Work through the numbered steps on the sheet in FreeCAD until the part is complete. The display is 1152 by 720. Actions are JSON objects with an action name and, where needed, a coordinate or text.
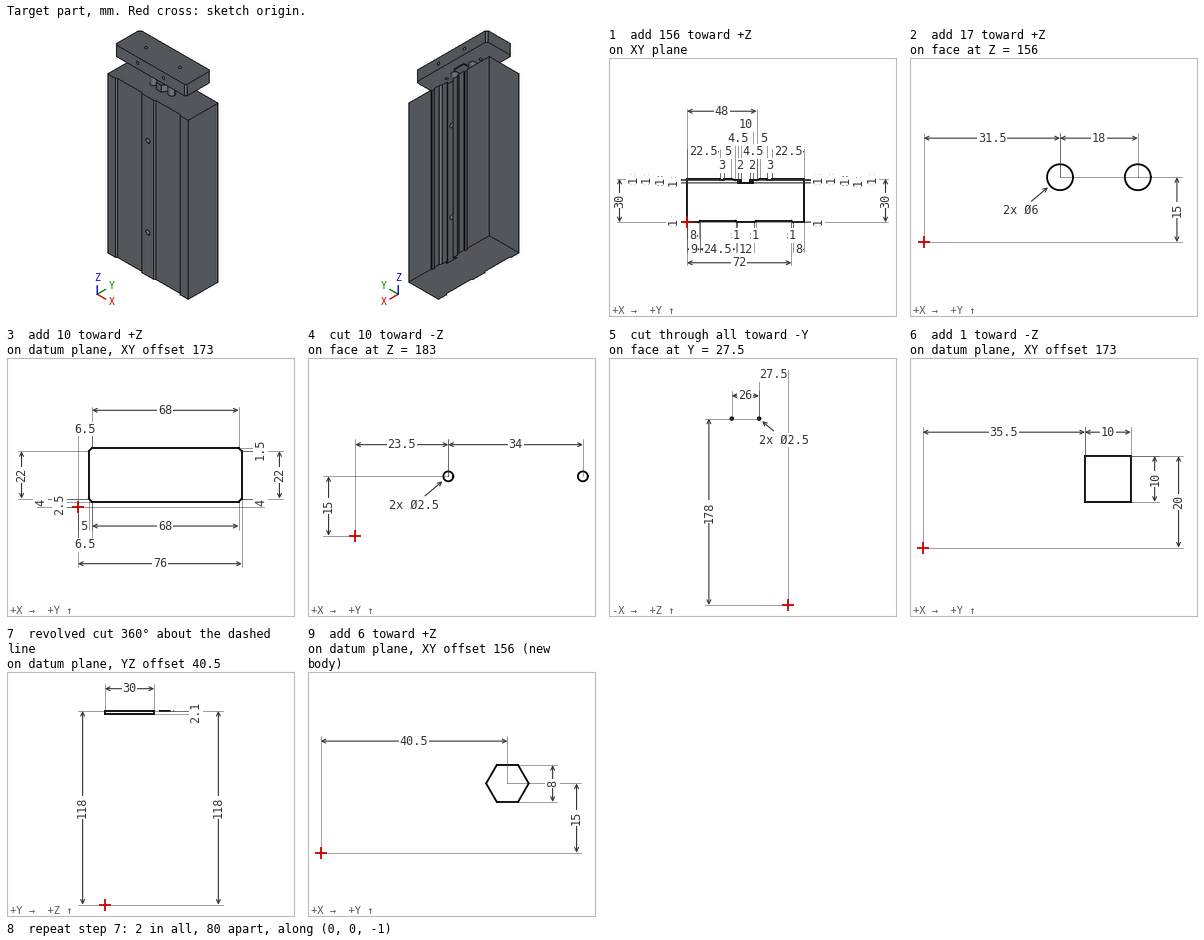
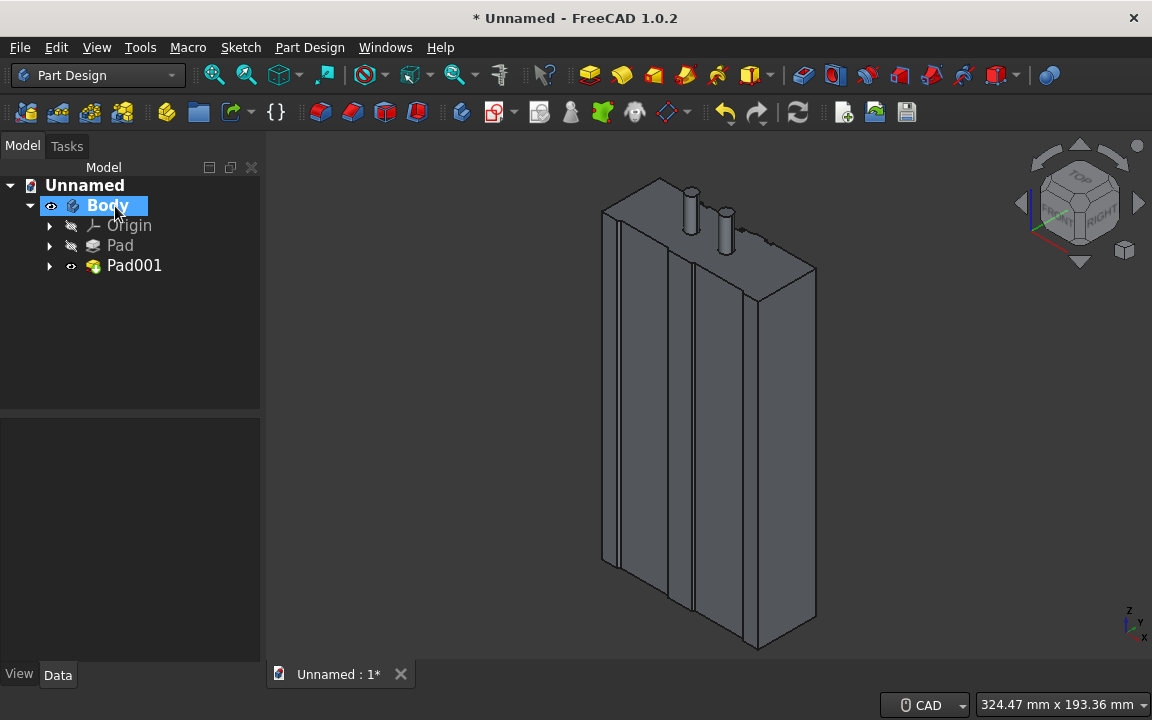
{"action": "key", "text": "2"}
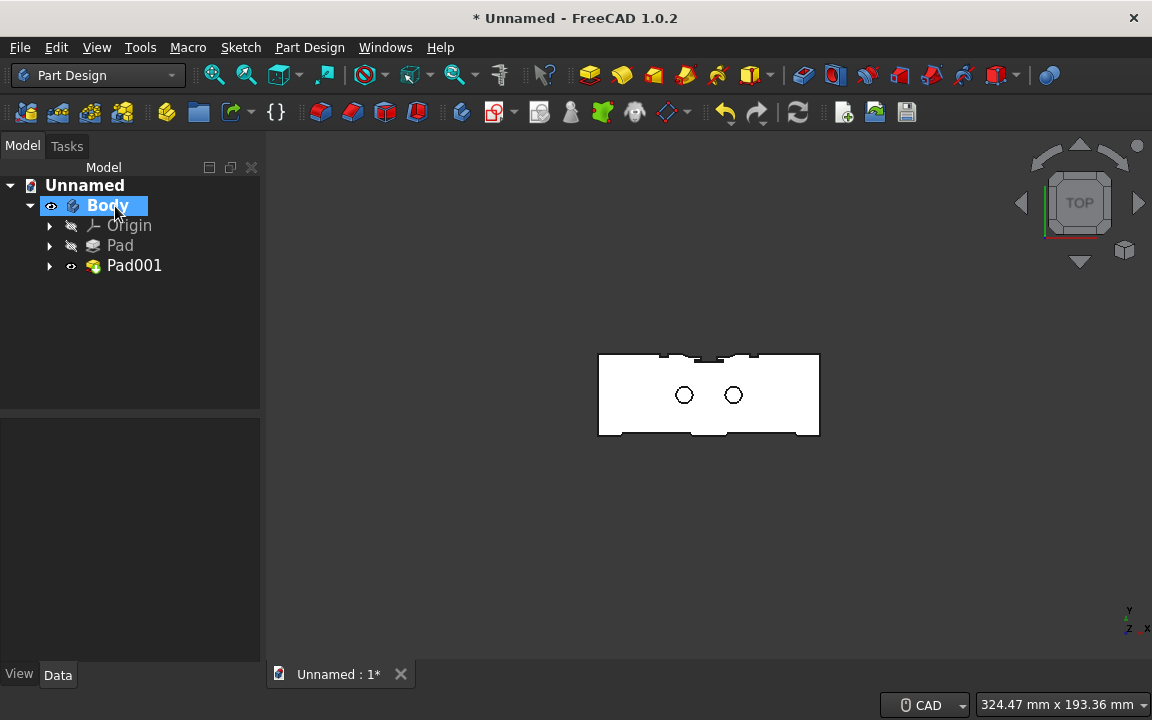
{"action": "key", "text": "v f"}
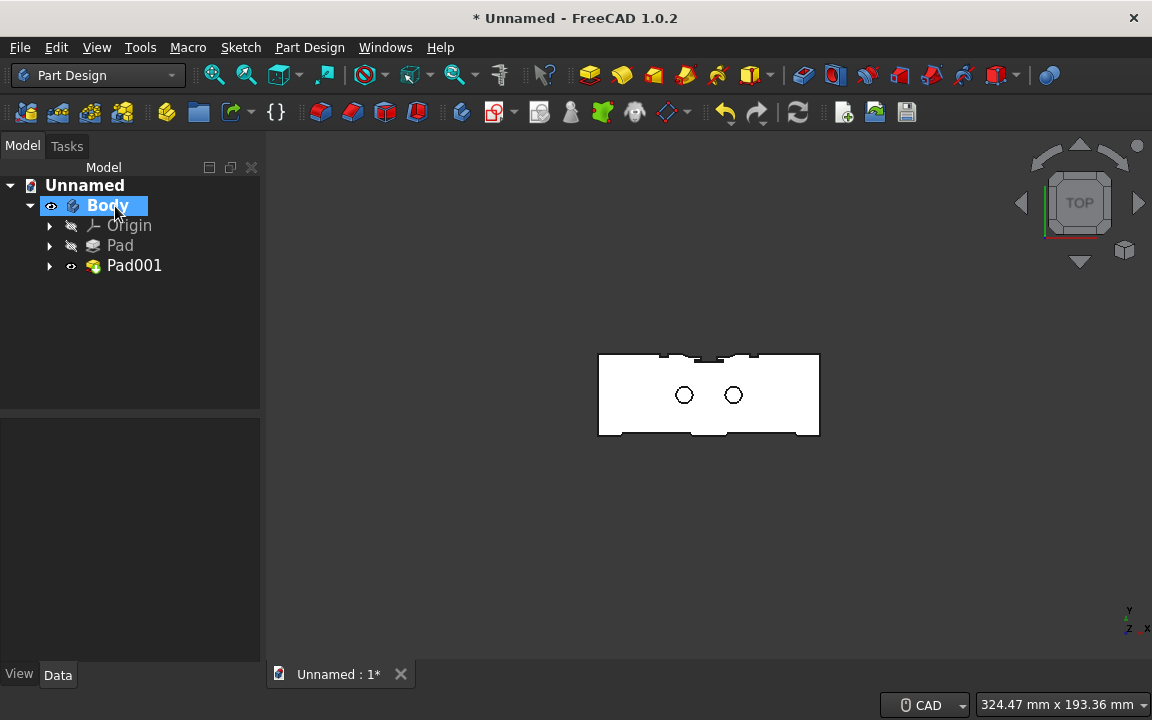
{"action": "key", "text": "1"}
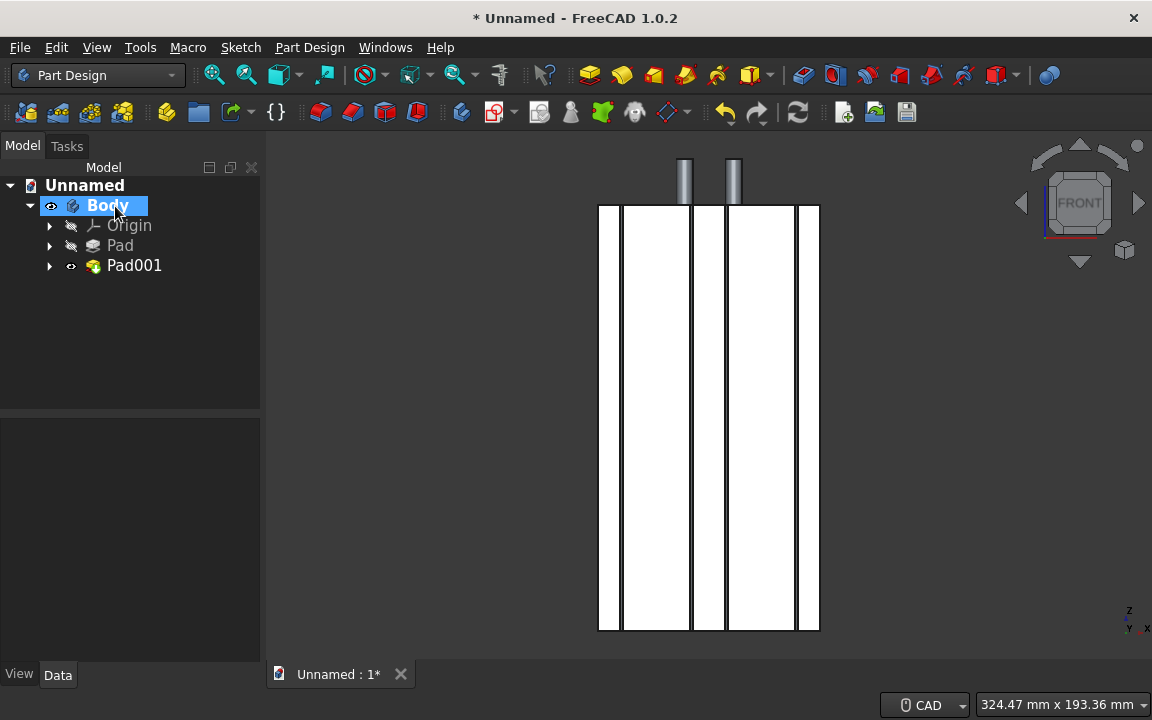
{"action": "left_click", "coordinate": [50, 226]}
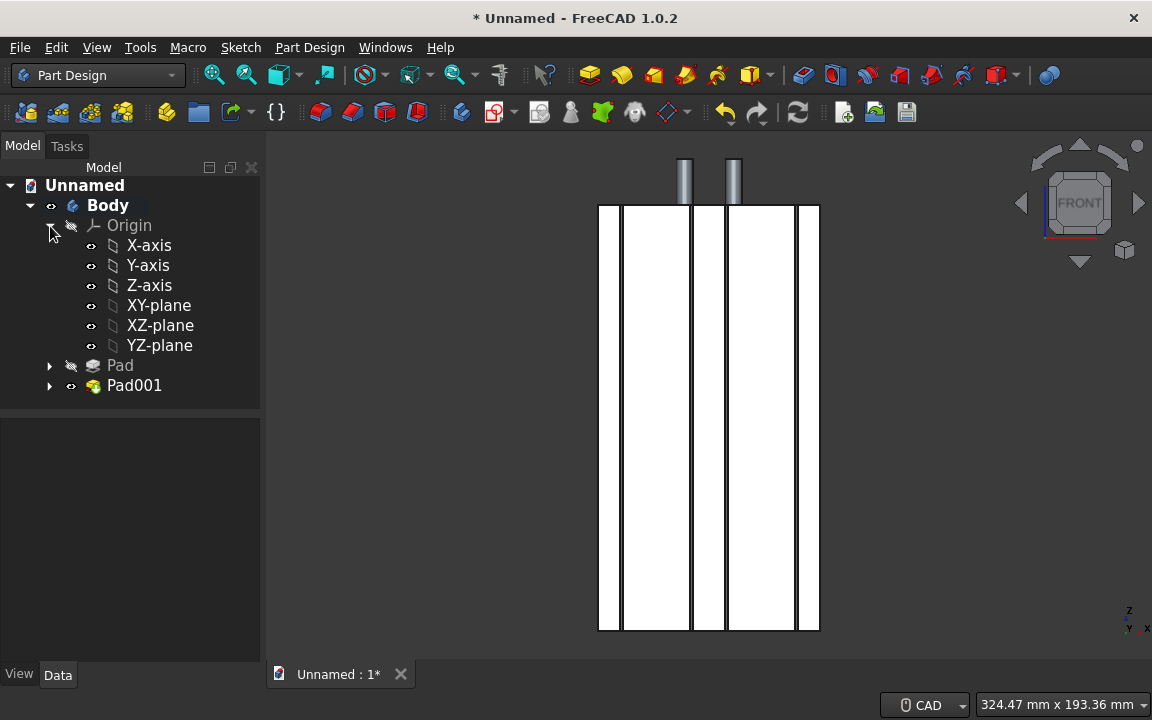
{"action": "left_click", "coordinate": [136, 306]}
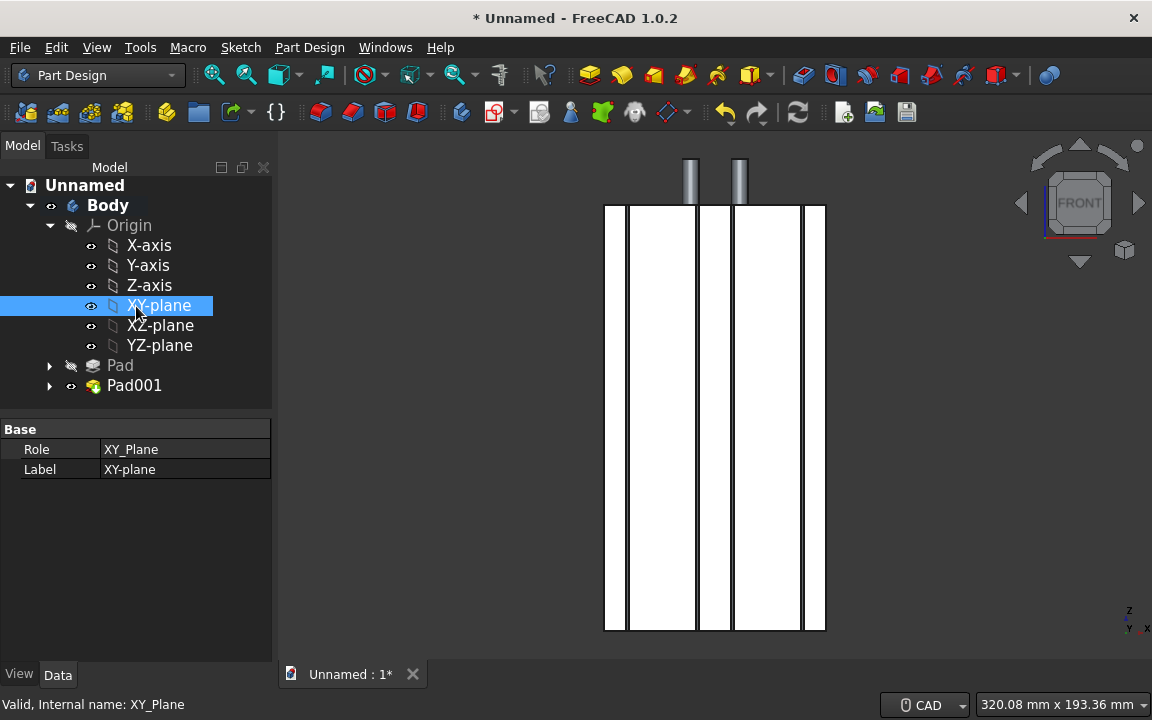
{"action": "left_click", "coordinate": [668, 112]}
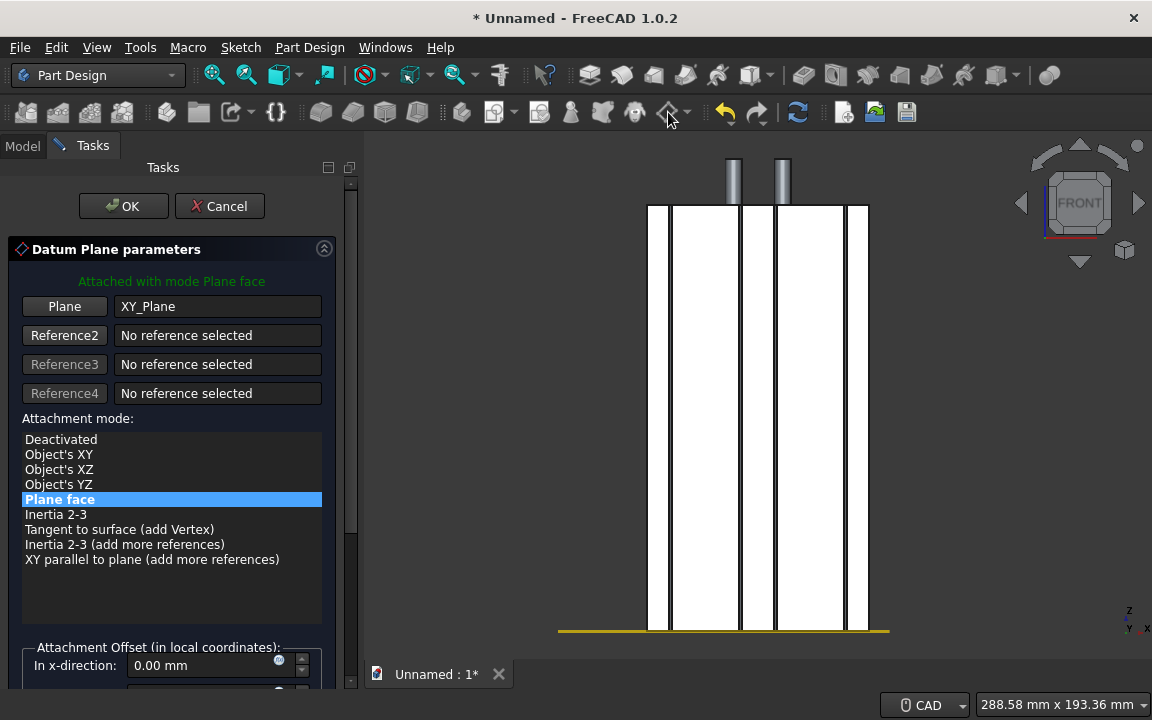
{"action": "scroll", "coordinate": [351, 432], "scroll_direction": "down", "scroll_amount": 2}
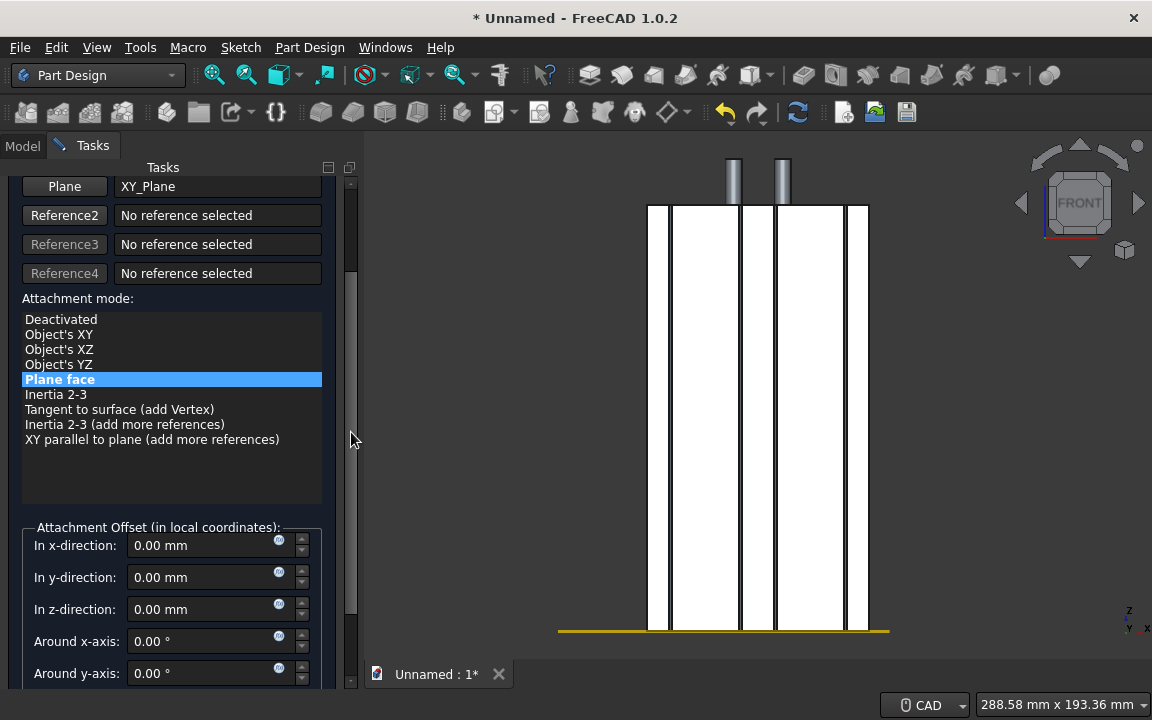
{"action": "triple_click", "coordinate": [210, 609]}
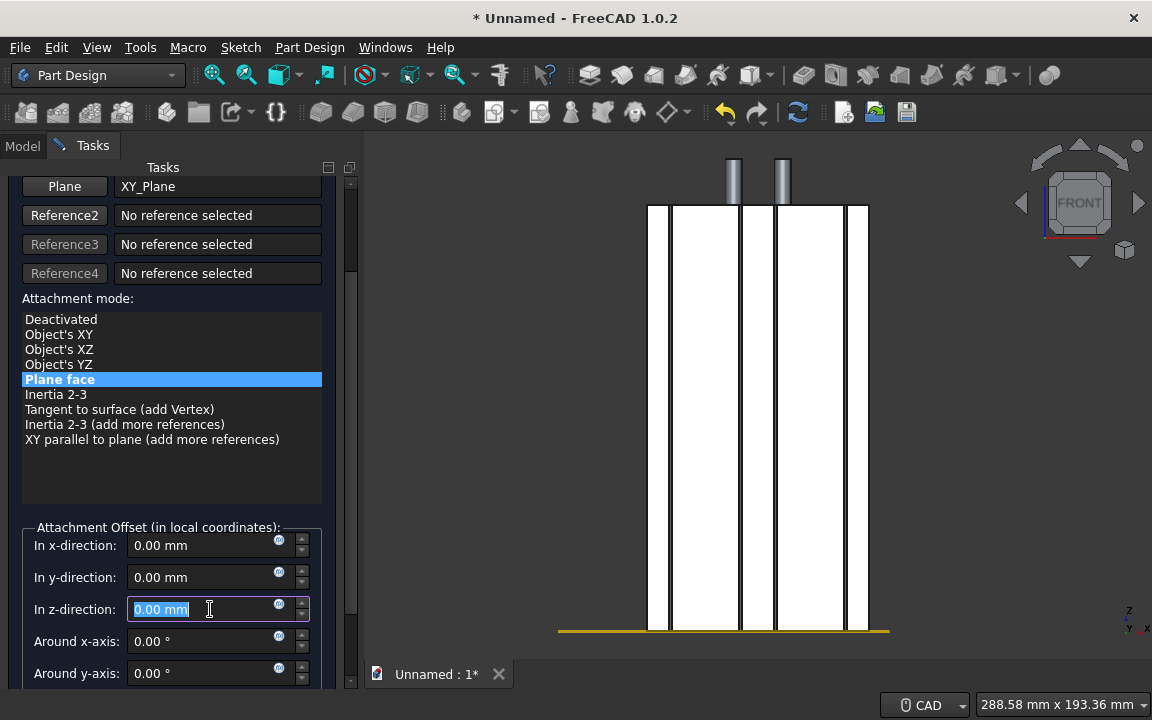
{"action": "type", "text": "173"}
{"action": "key", "text": "Tab"}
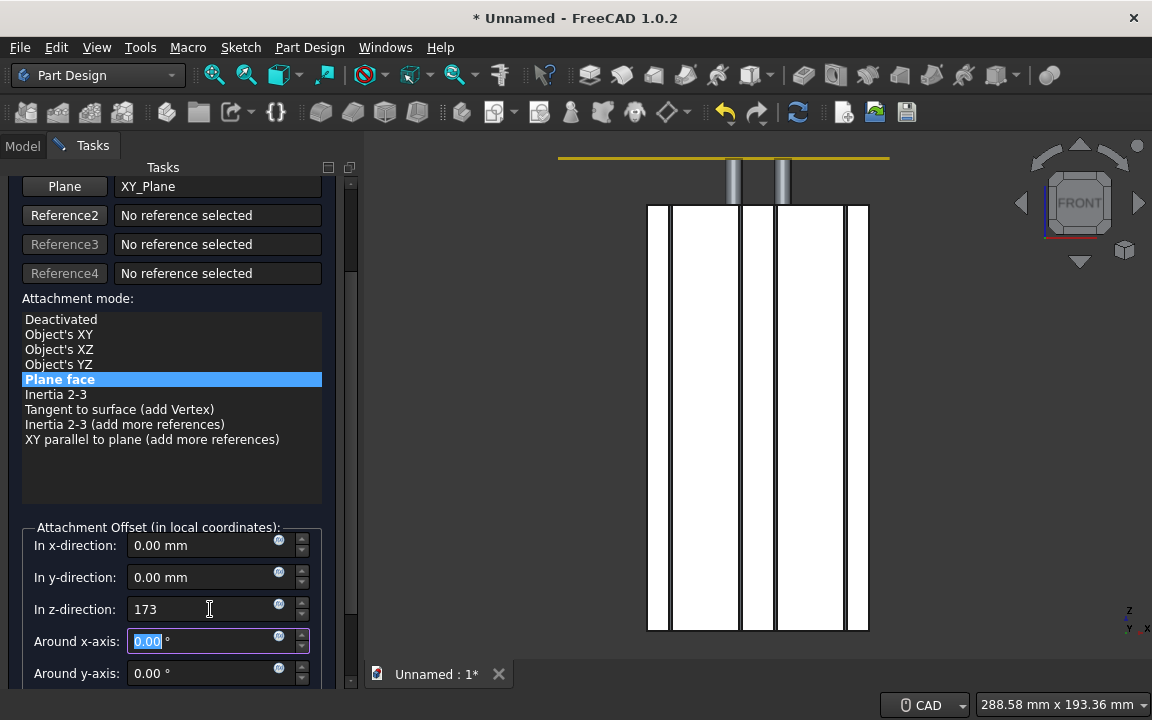
{"action": "scroll", "coordinate": [351, 432], "scroll_direction": "up", "scroll_amount": 3}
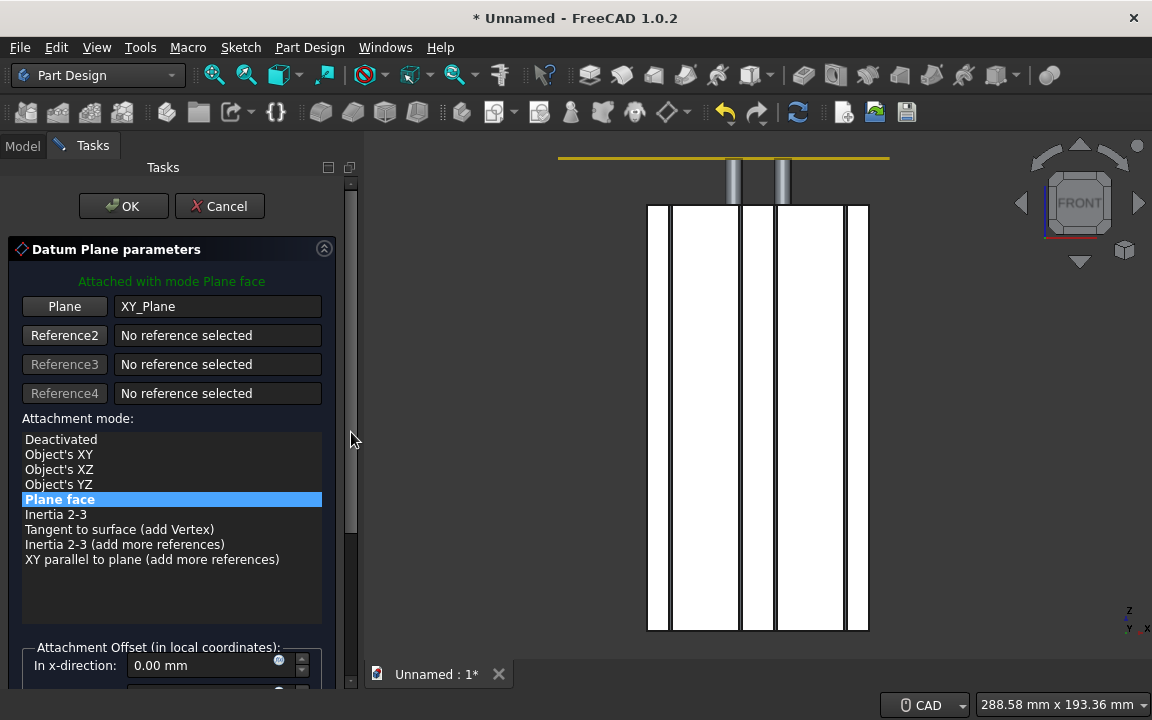
{"action": "left_click", "coordinate": [124, 206]}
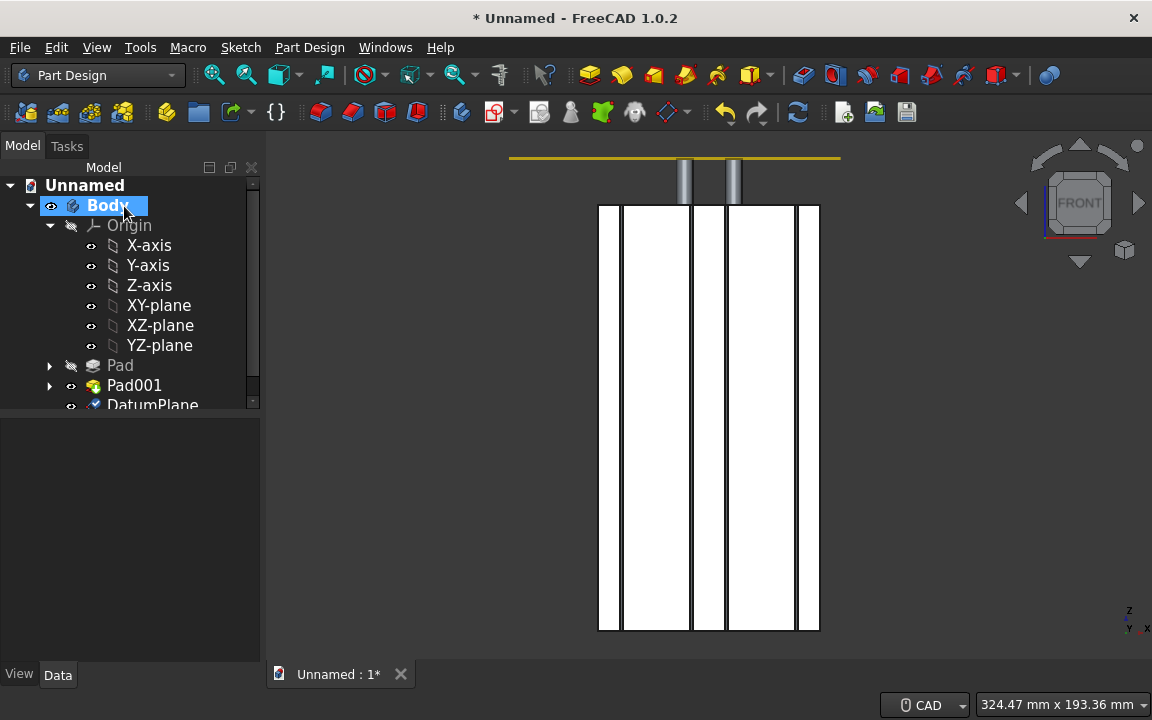
{"action": "left_click", "coordinate": [116, 406]}